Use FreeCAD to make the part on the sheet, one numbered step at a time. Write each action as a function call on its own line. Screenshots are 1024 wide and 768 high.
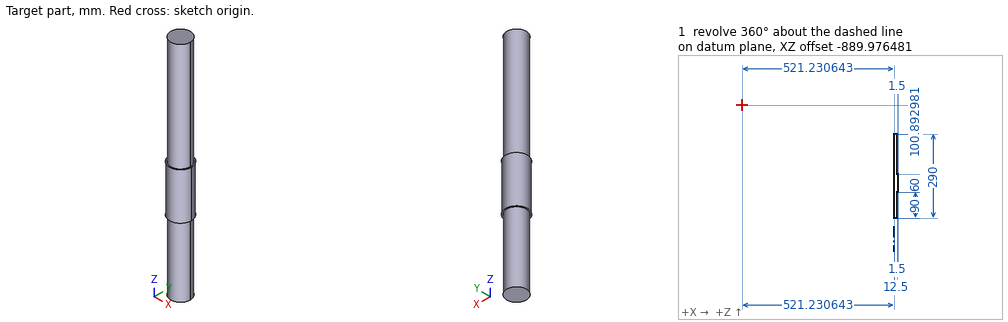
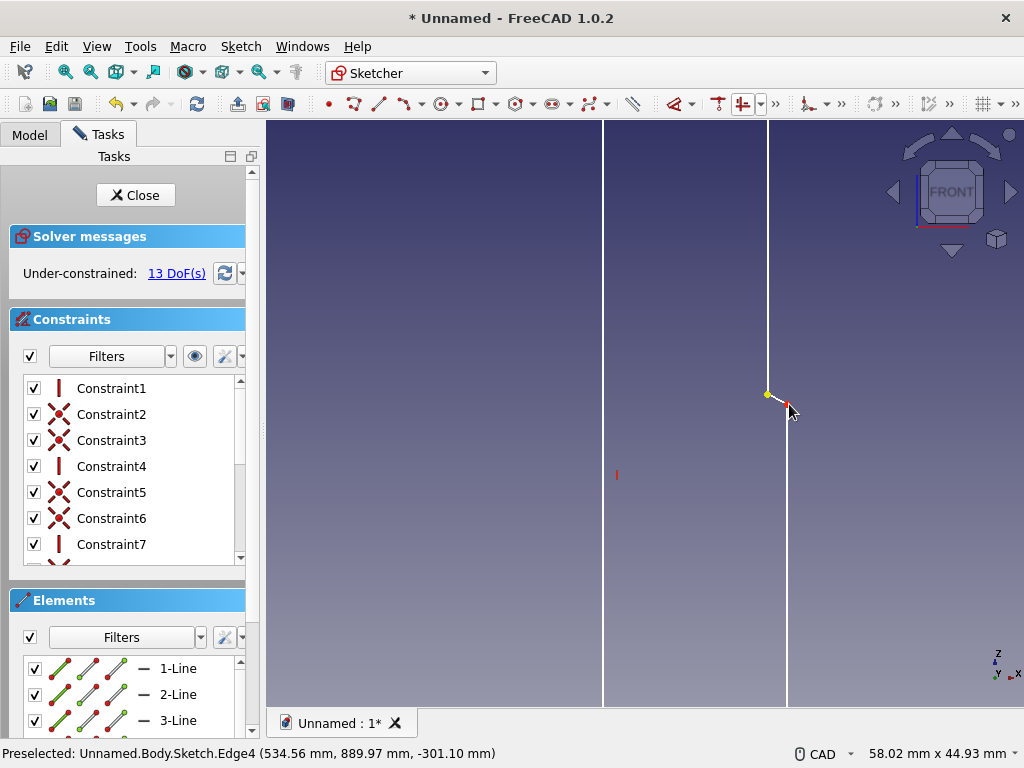
click(778, 399)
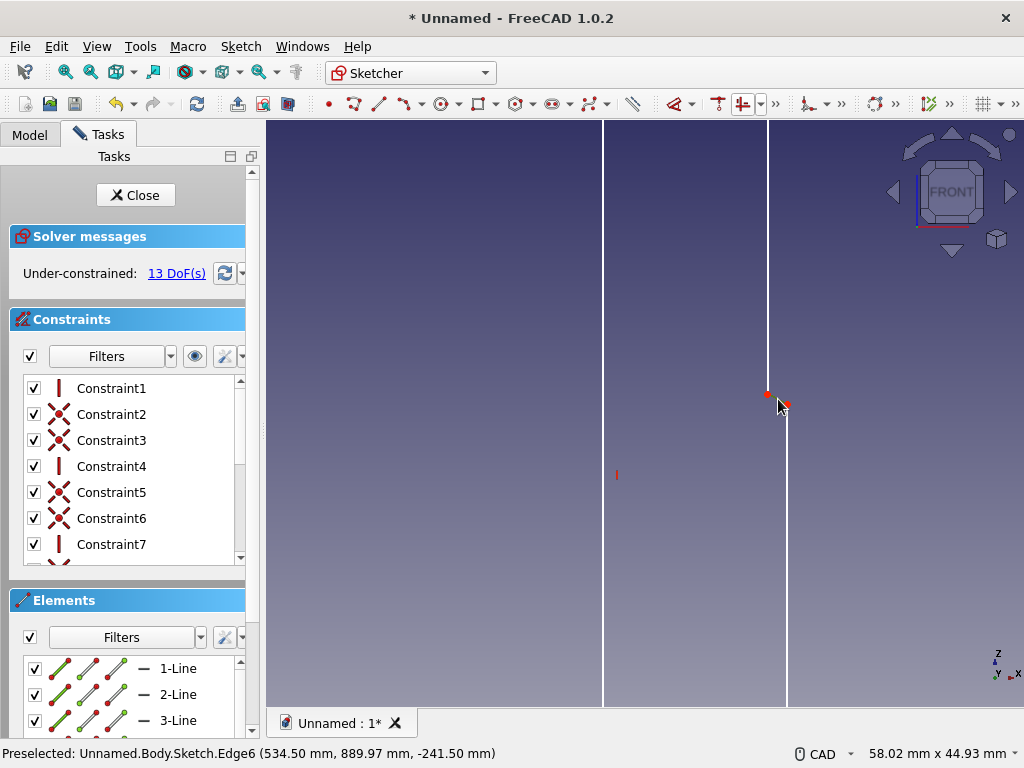
click(760, 104)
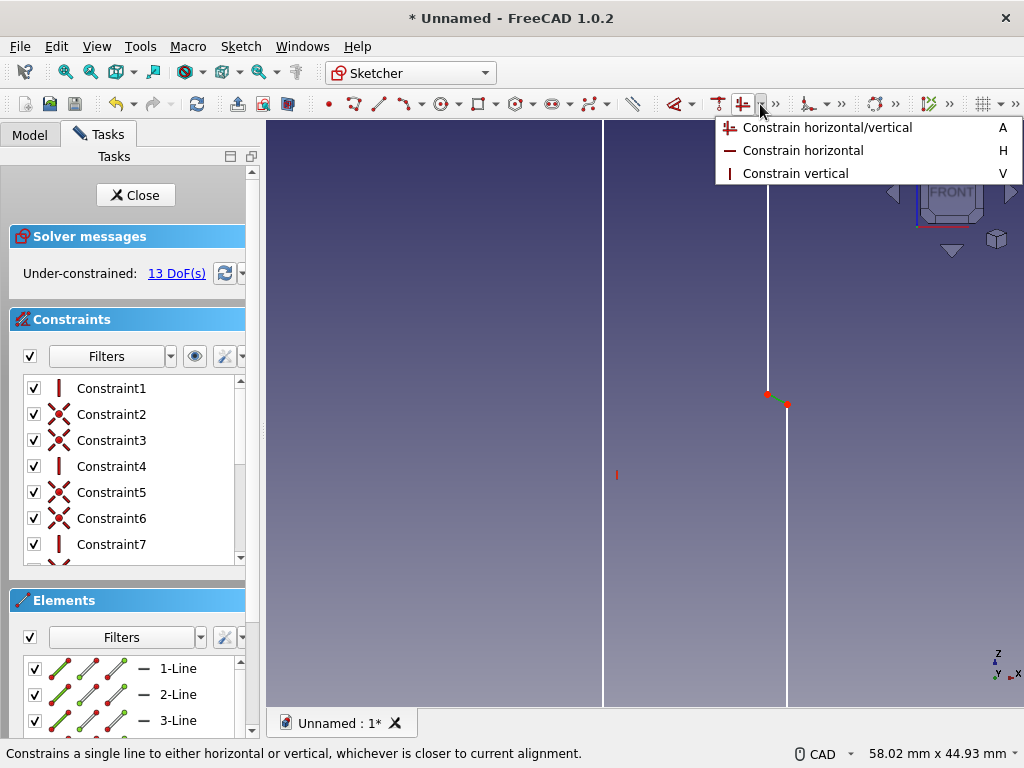
click(869, 150)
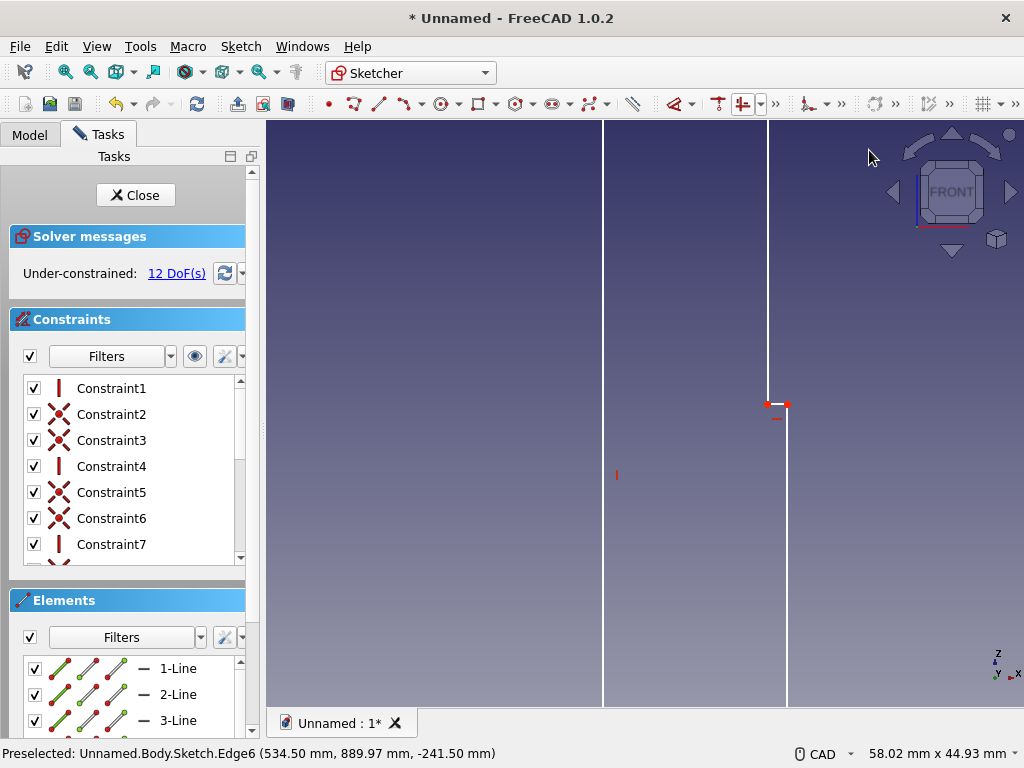
scroll(789, 404, down, 14)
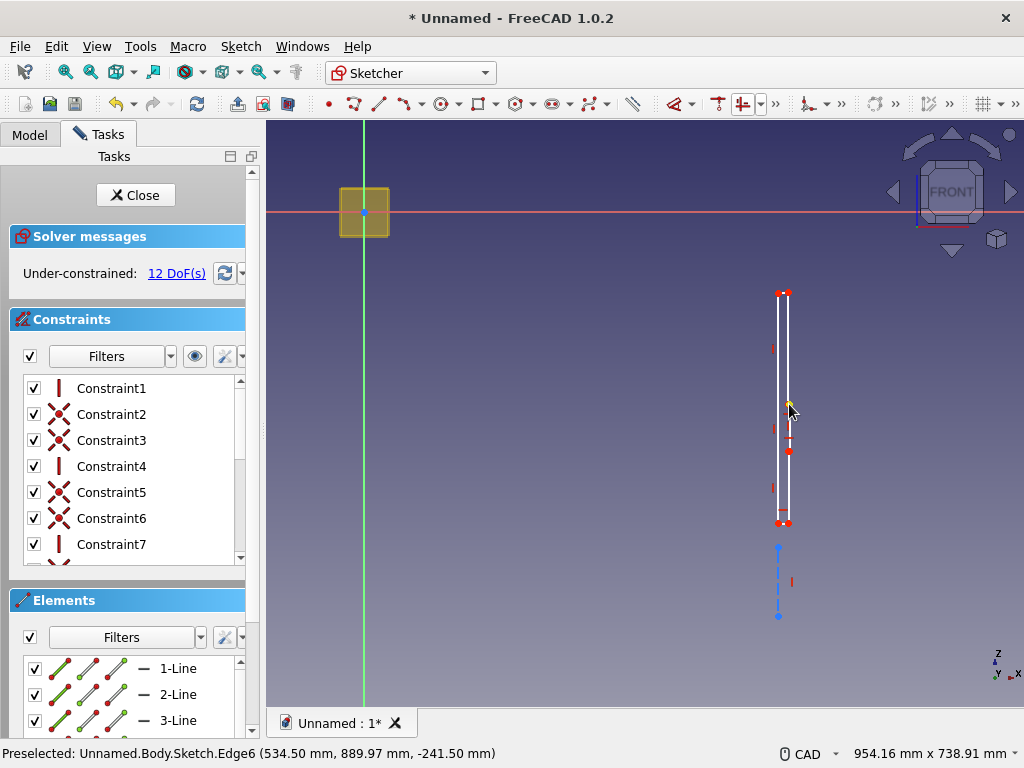
scroll(785, 293, up, 8)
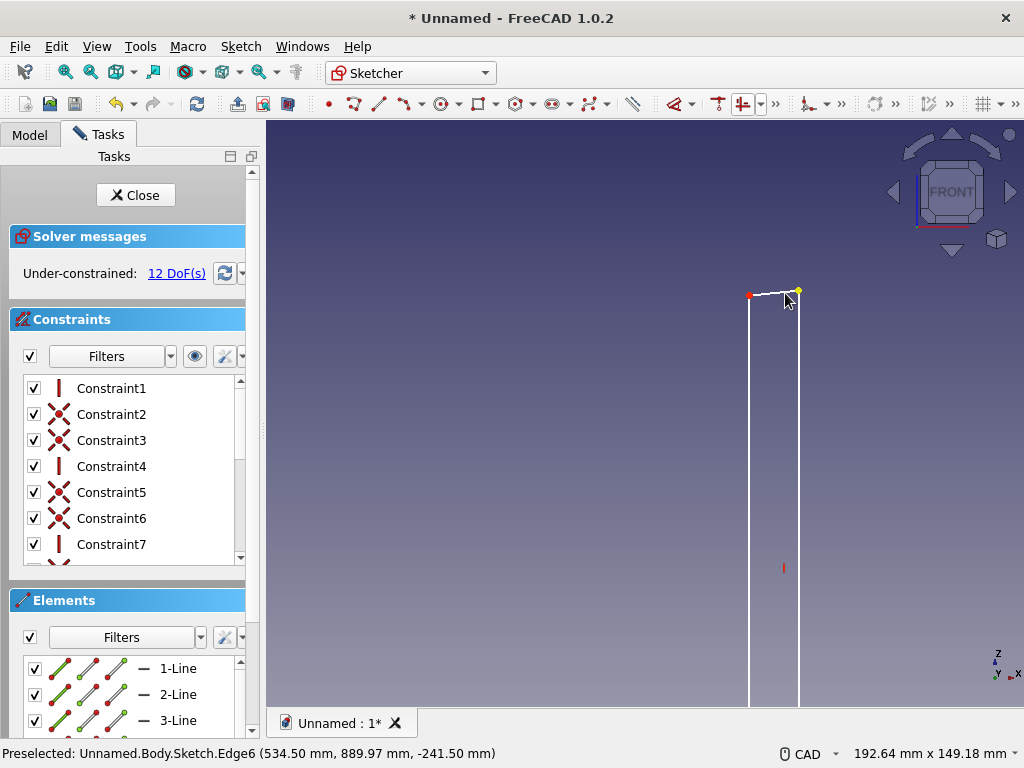
click(784, 292)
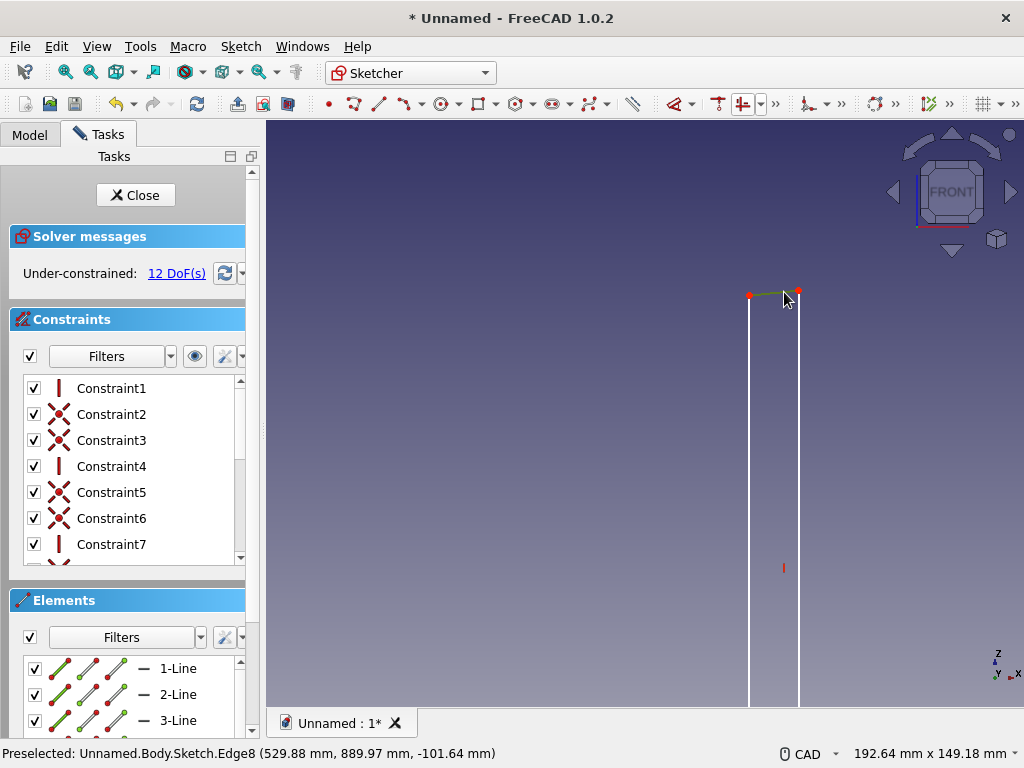
click(760, 104)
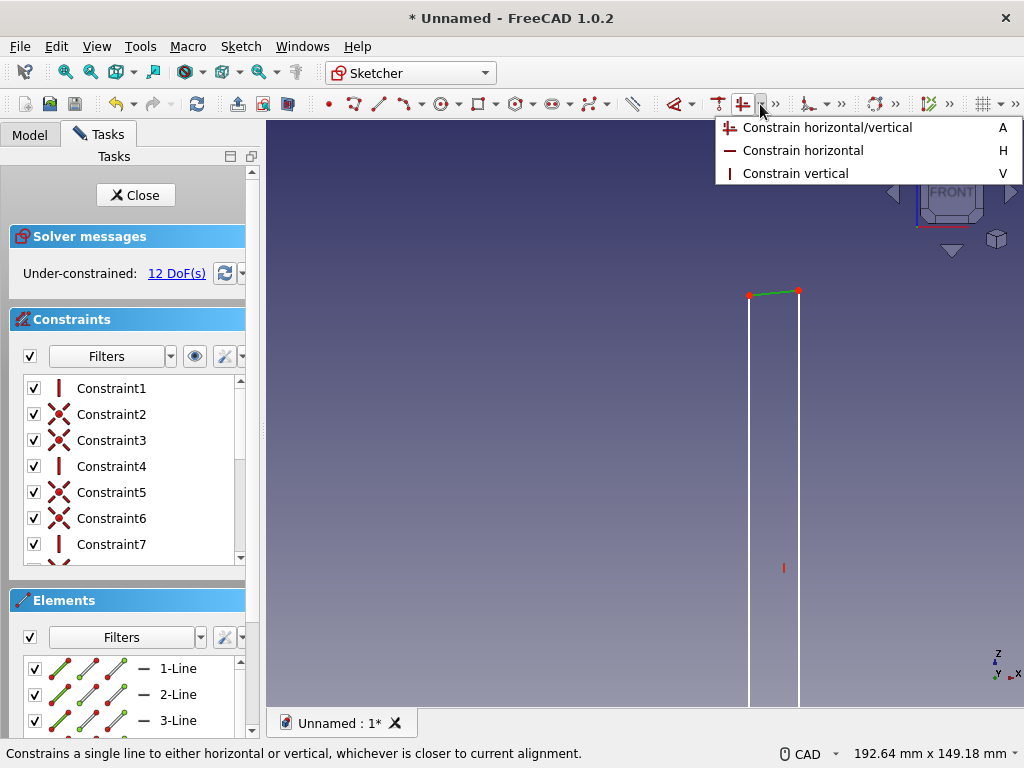
click(869, 150)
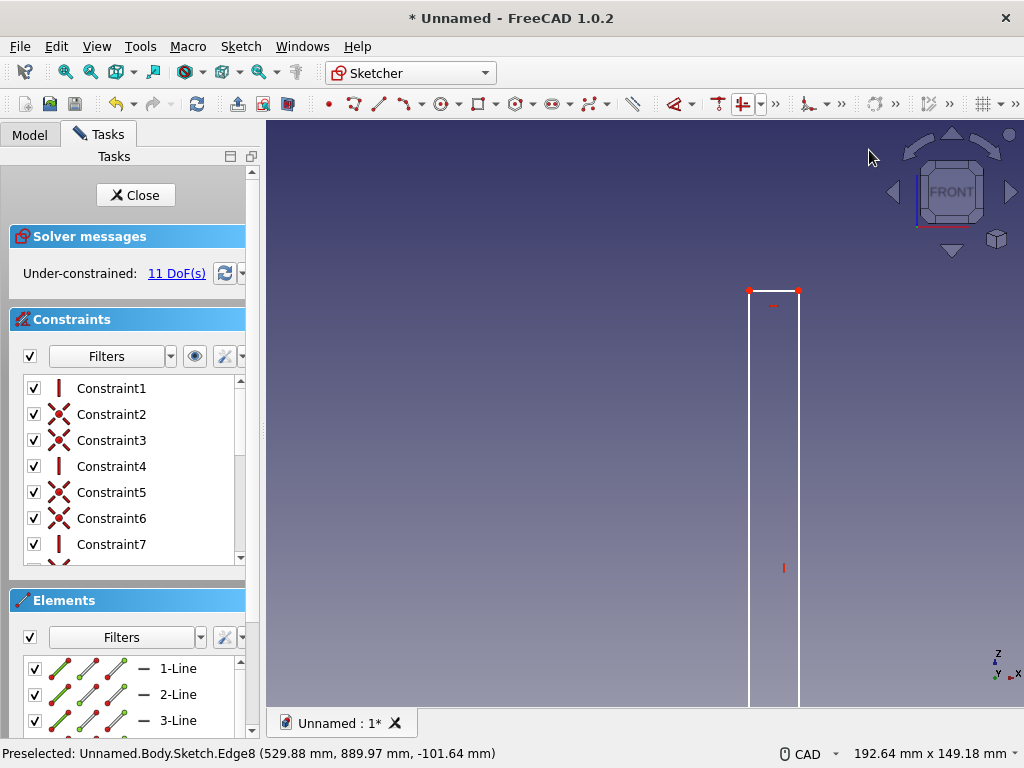
scroll(785, 293, down, 8)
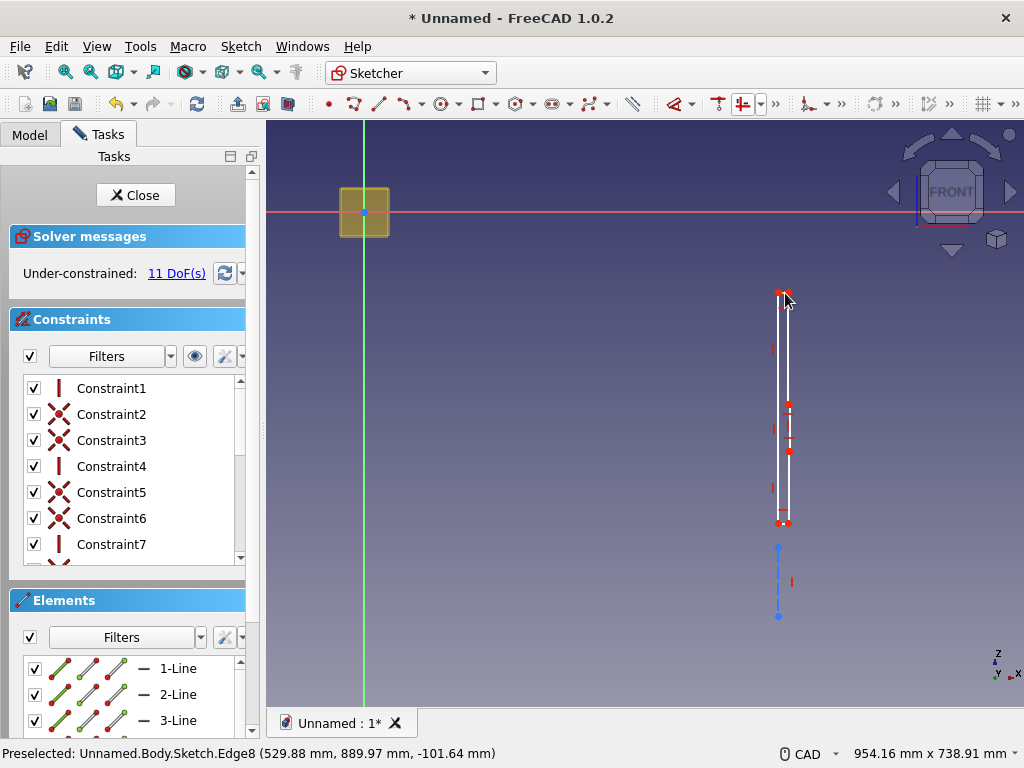
scroll(789, 502, up, 2)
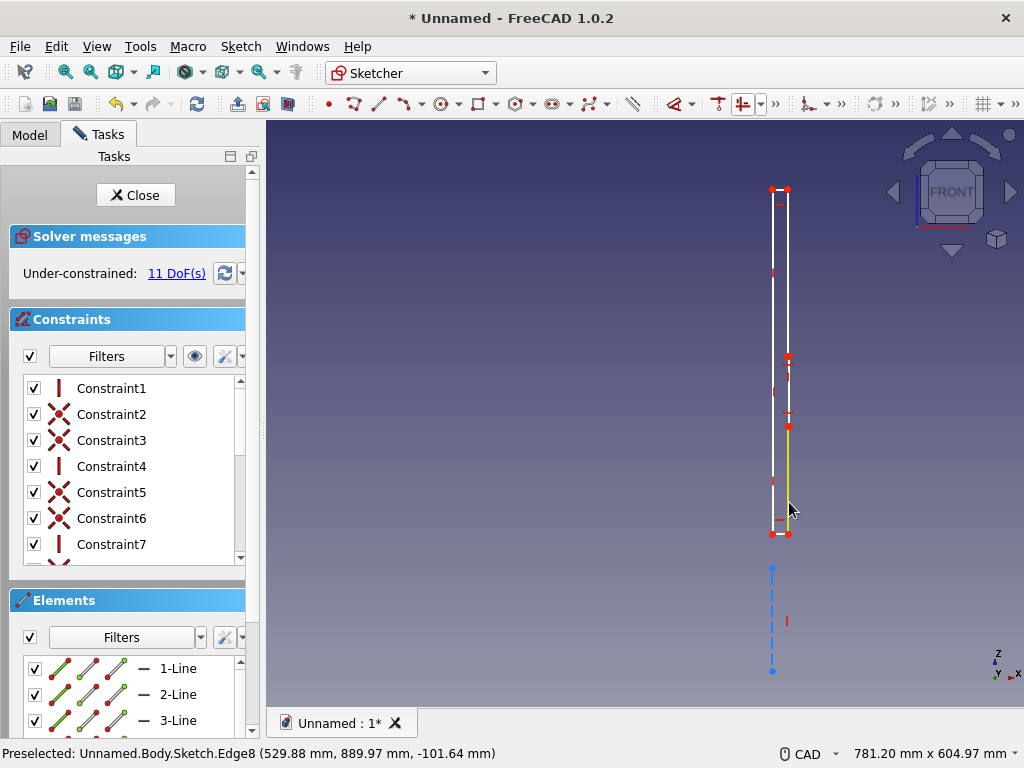
click(788, 502)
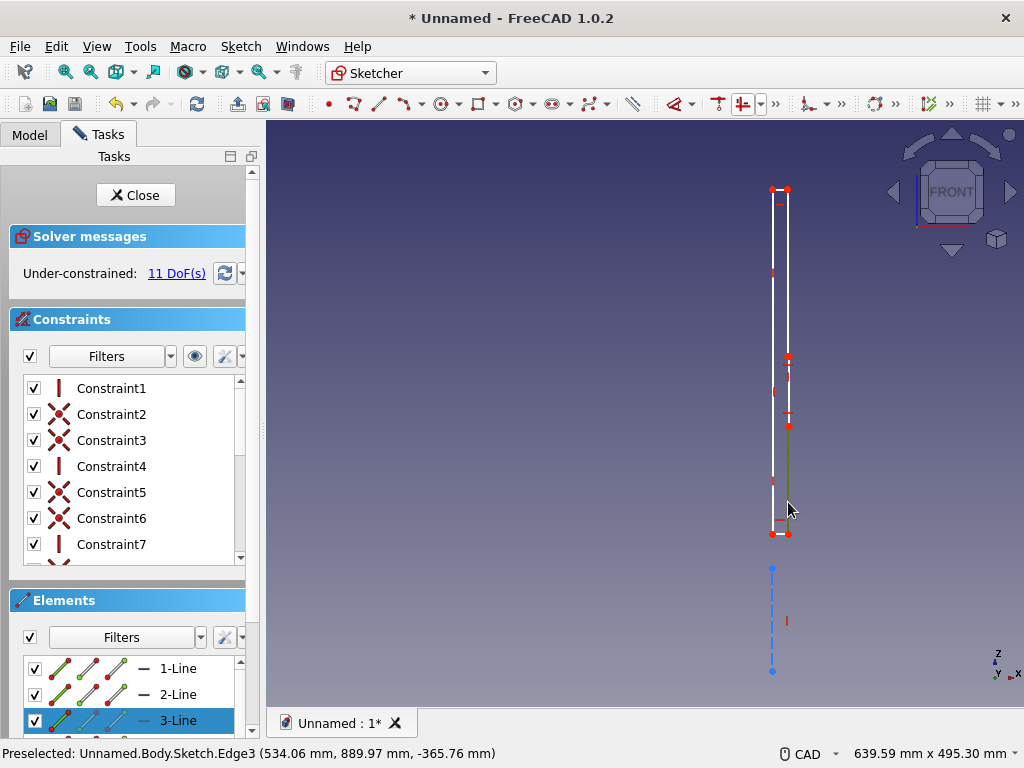
click(692, 104)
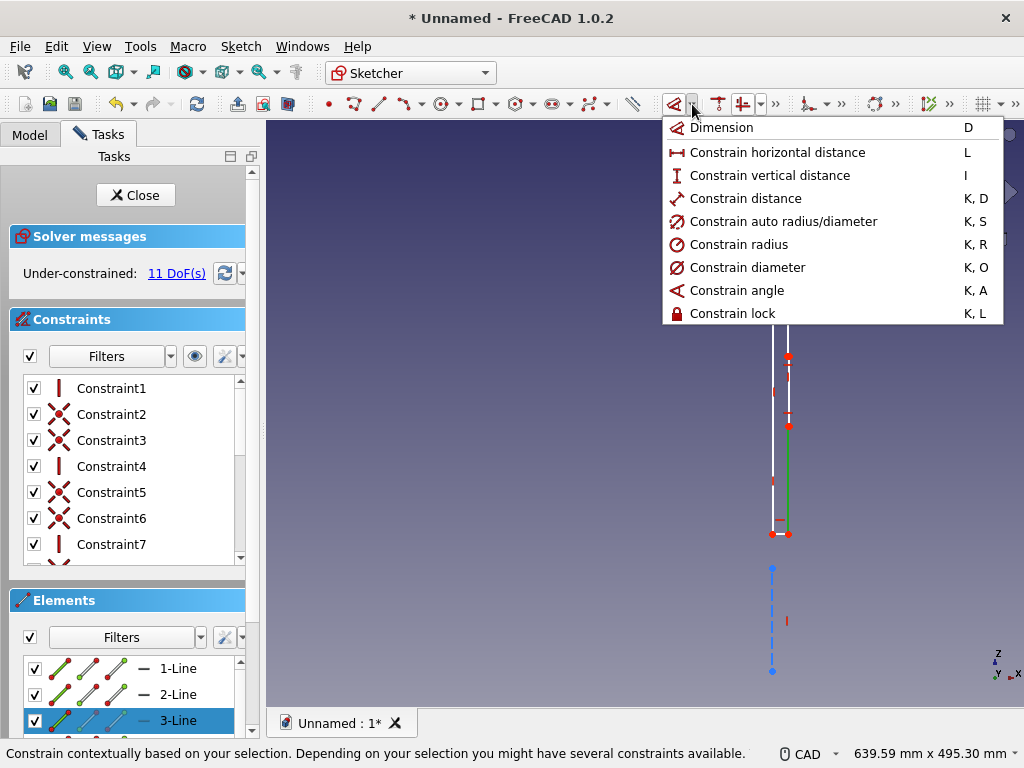
click(833, 176)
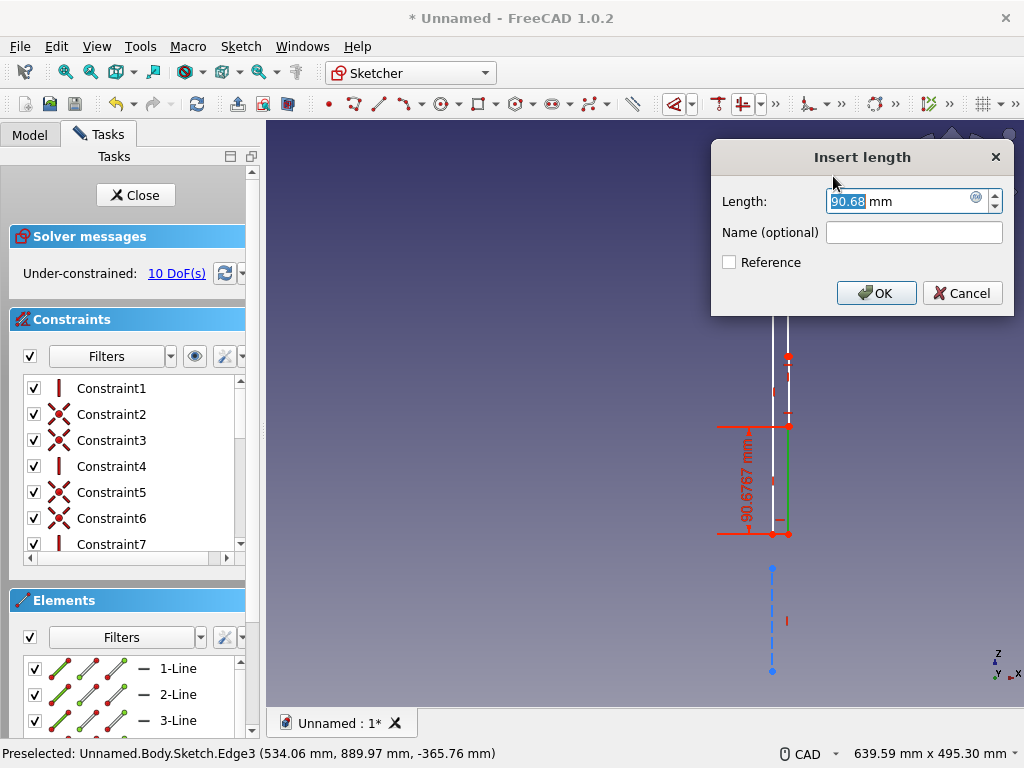
text(90)
key(Return)